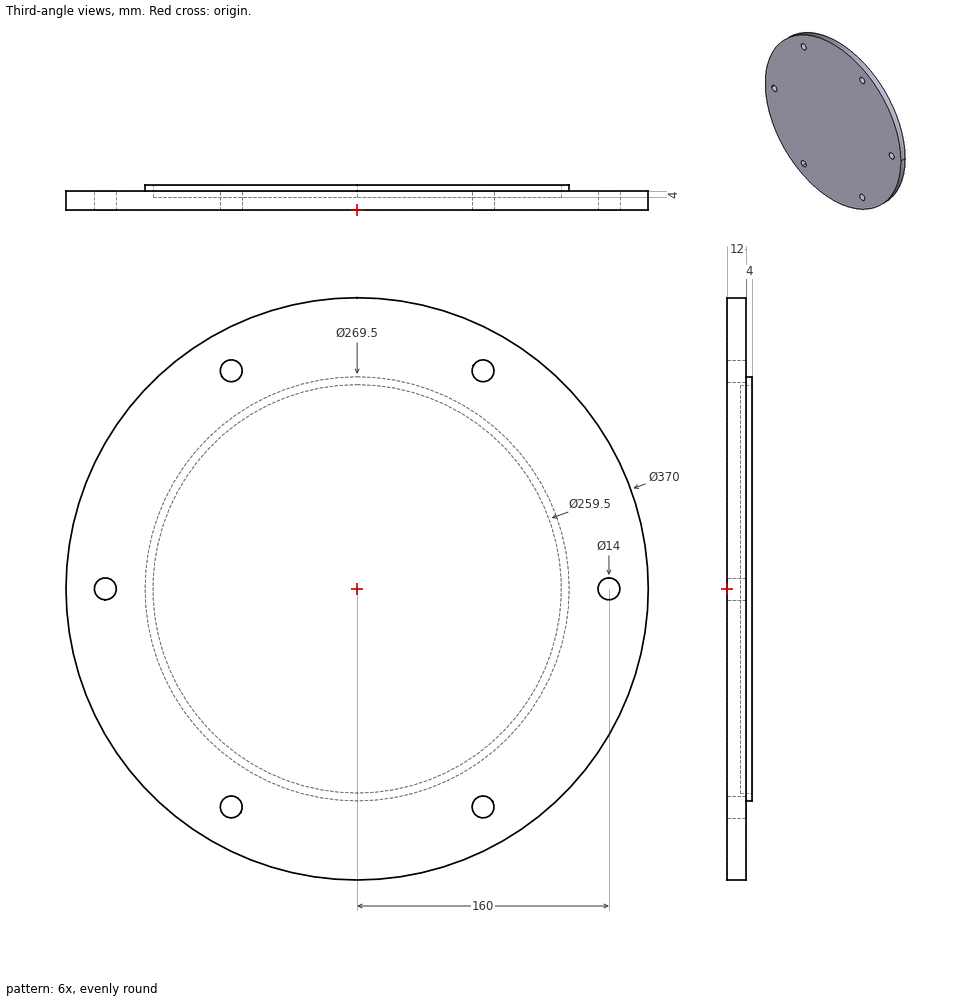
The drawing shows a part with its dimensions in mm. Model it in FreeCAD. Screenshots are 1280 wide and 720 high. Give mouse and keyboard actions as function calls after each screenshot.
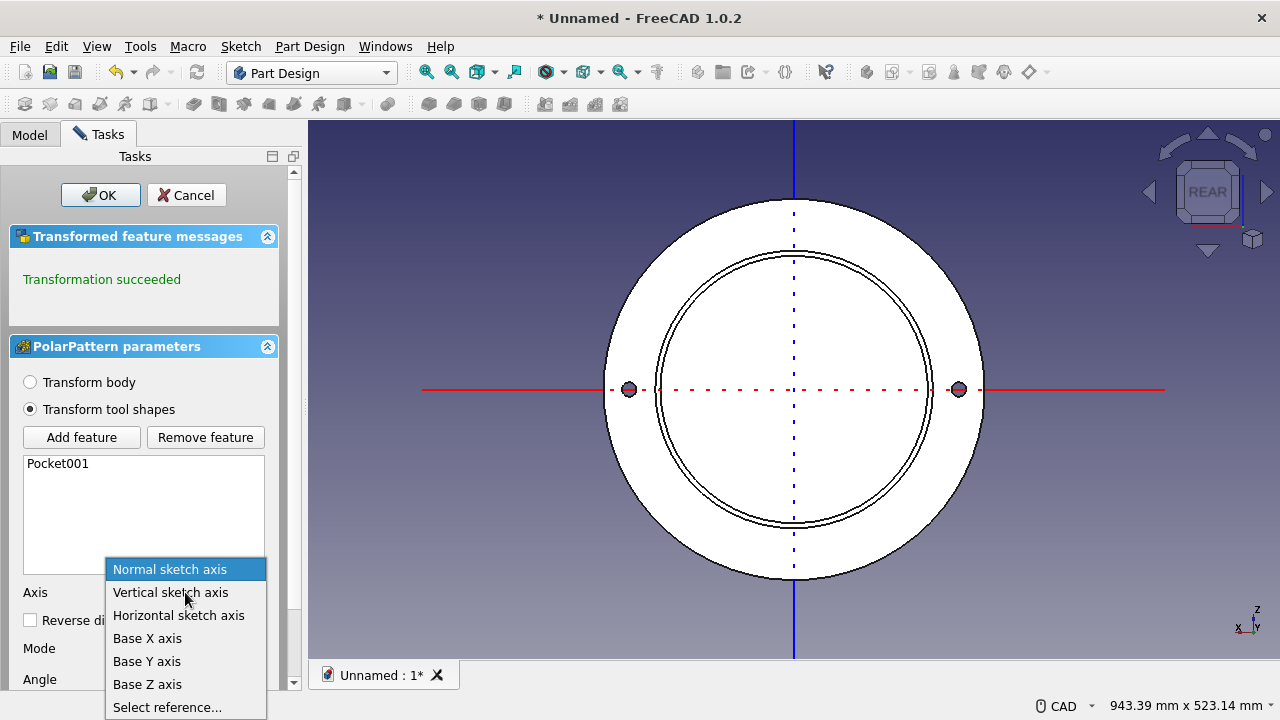
click(184, 662)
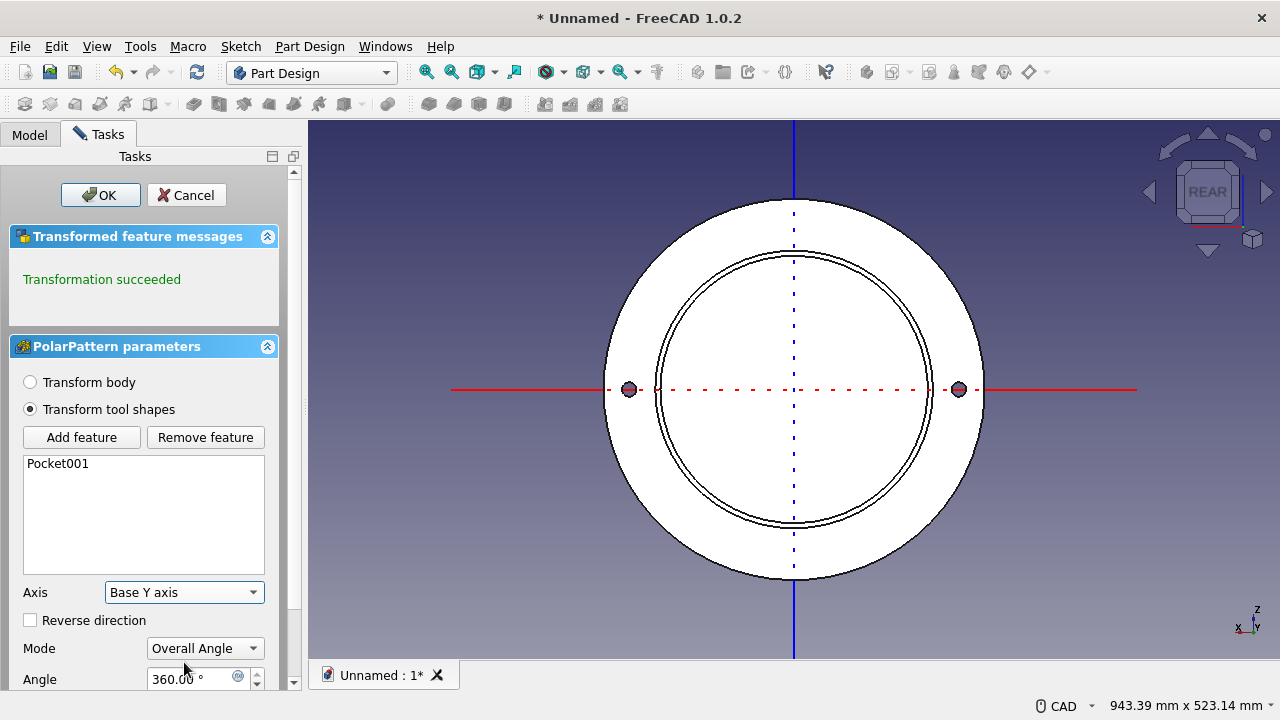
scroll(294, 428, down, 2)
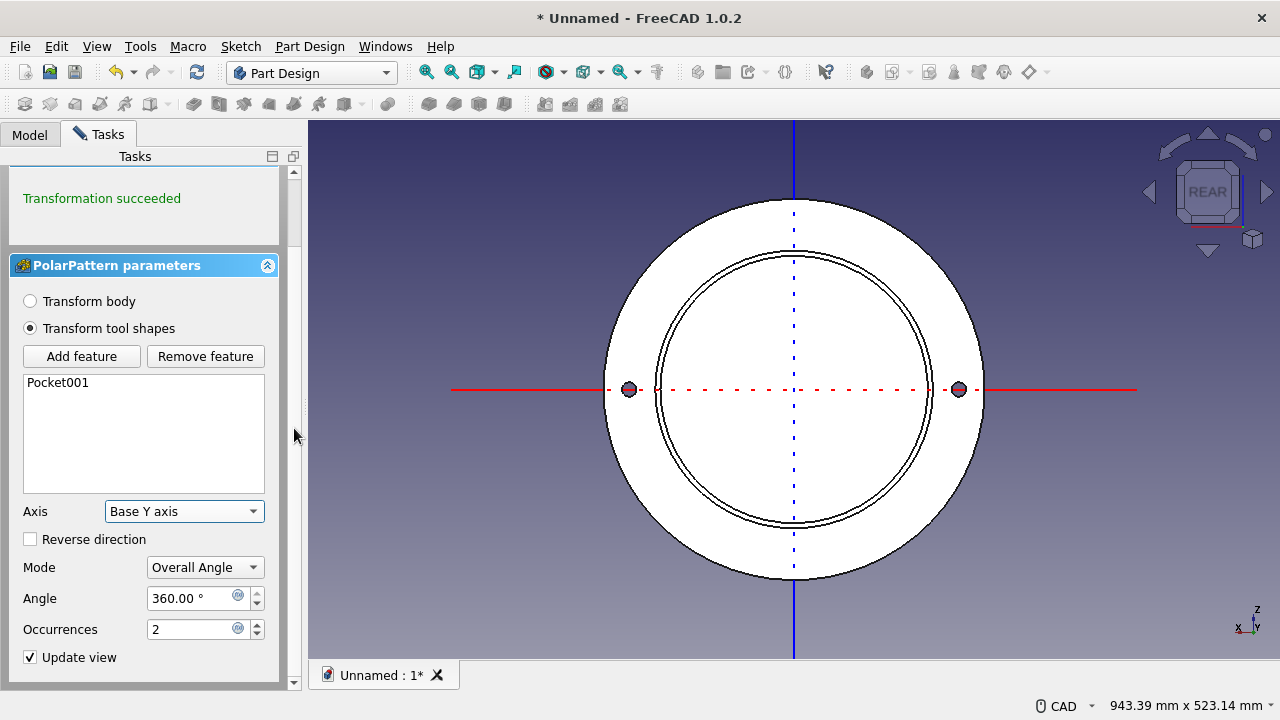
triple_click(199, 630)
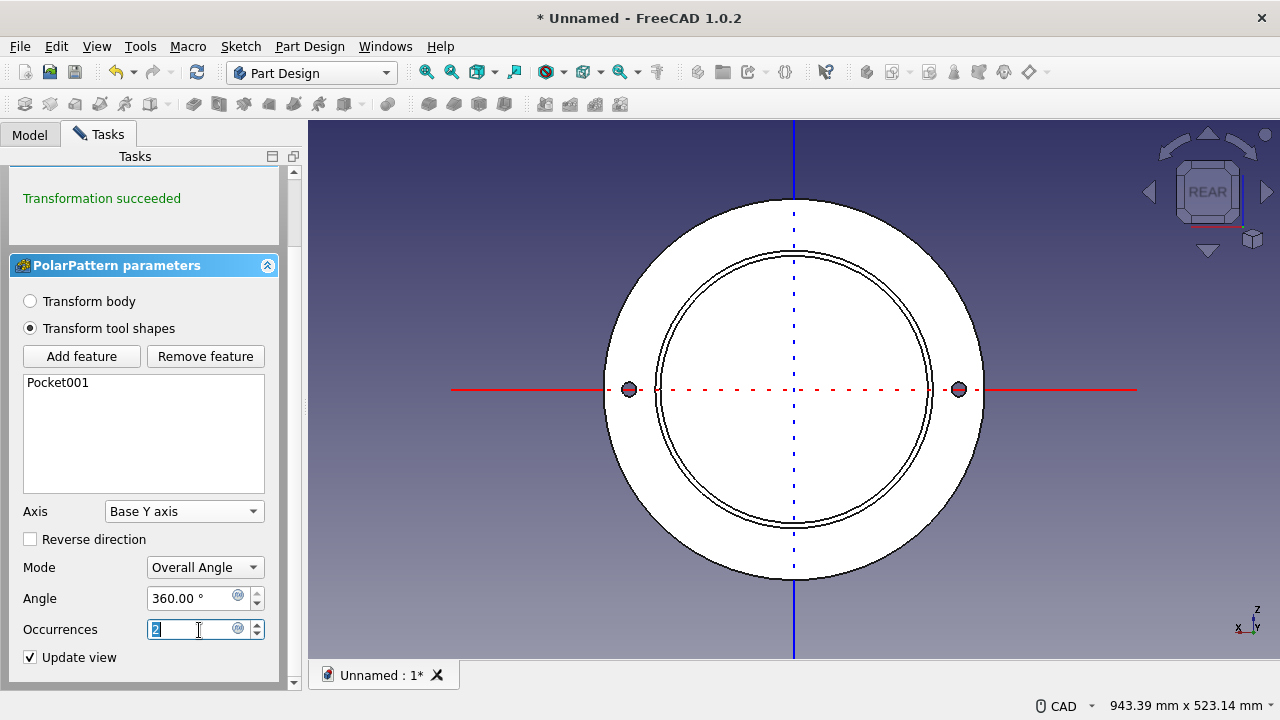
text(6)
key(Tab)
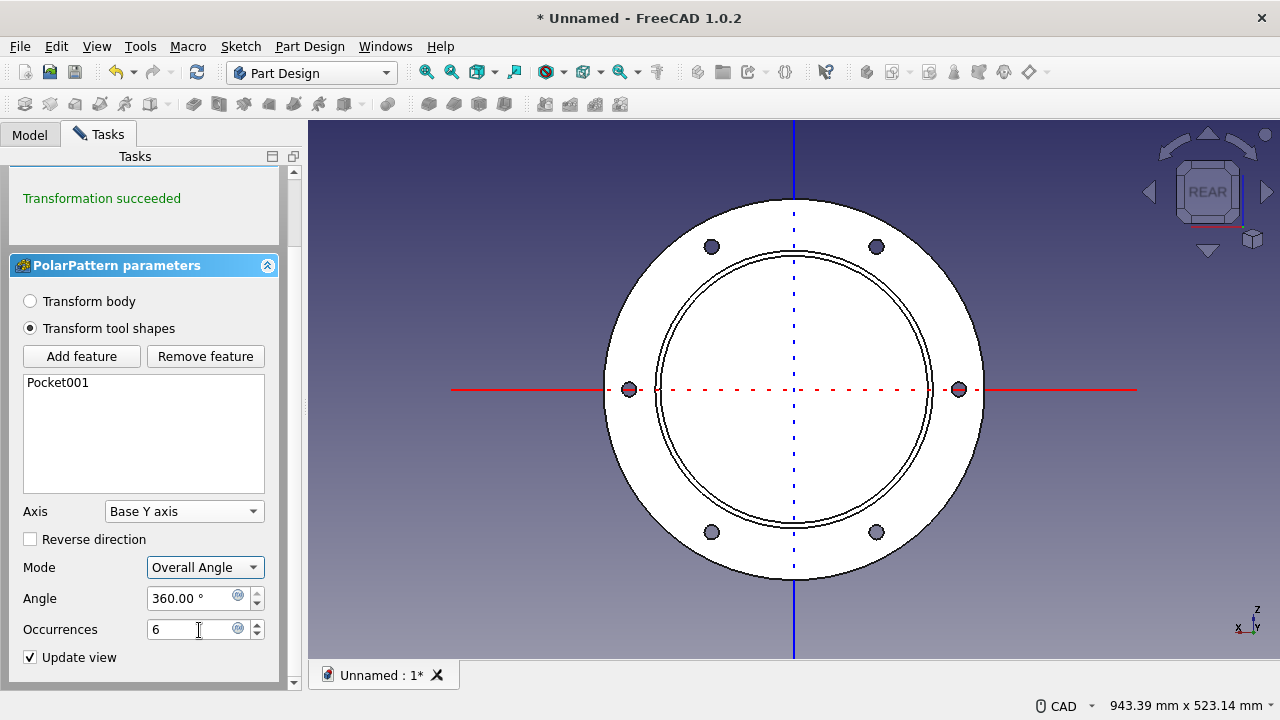
scroll(294, 428, up, 3)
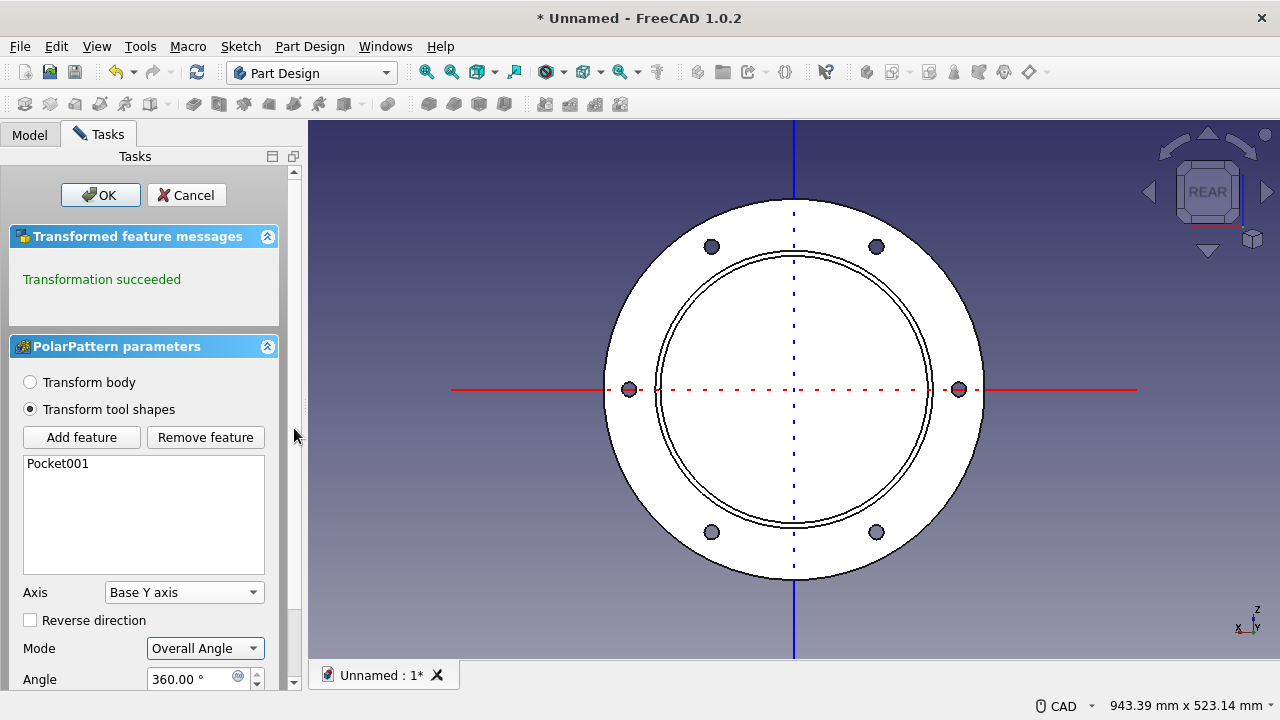
click(101, 195)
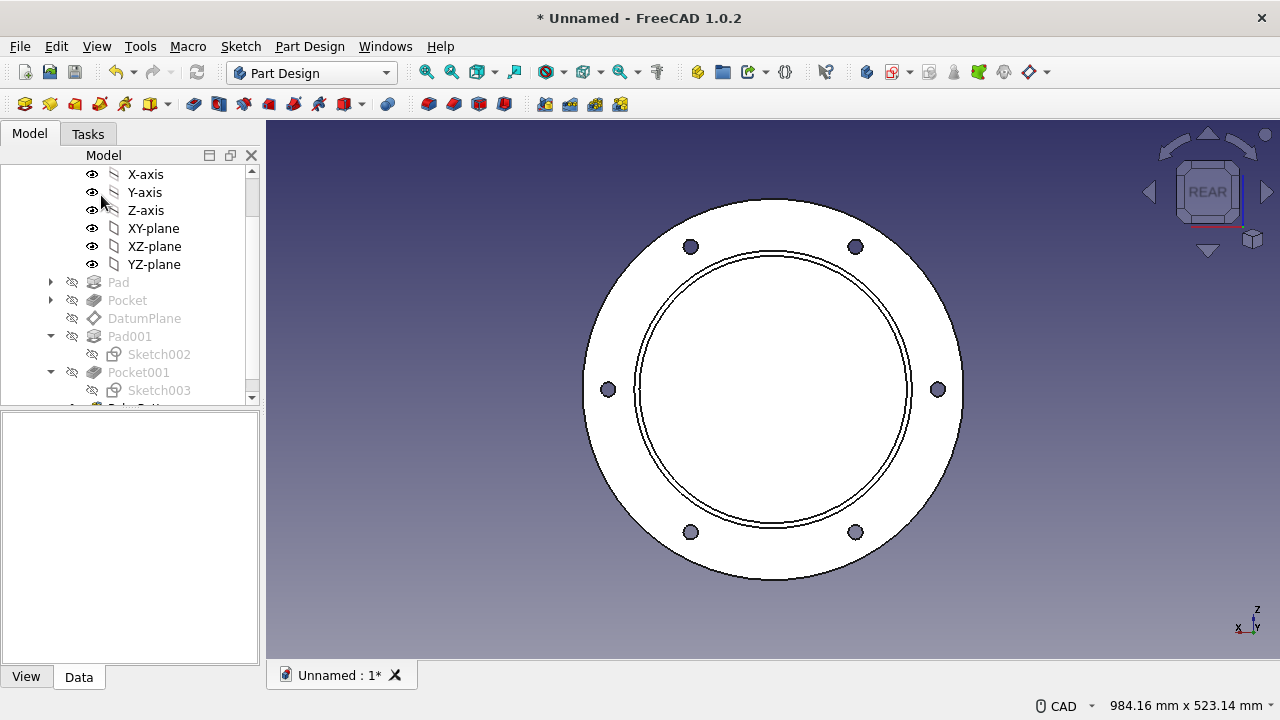
key(0)